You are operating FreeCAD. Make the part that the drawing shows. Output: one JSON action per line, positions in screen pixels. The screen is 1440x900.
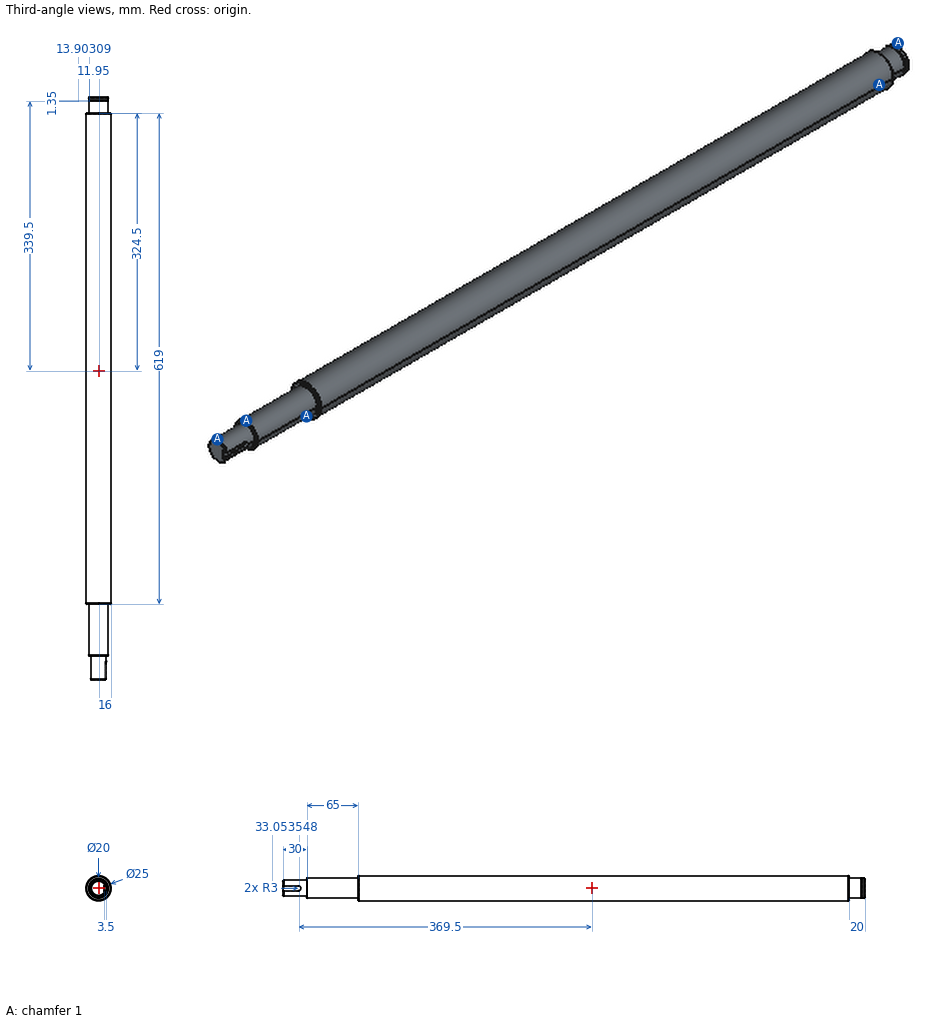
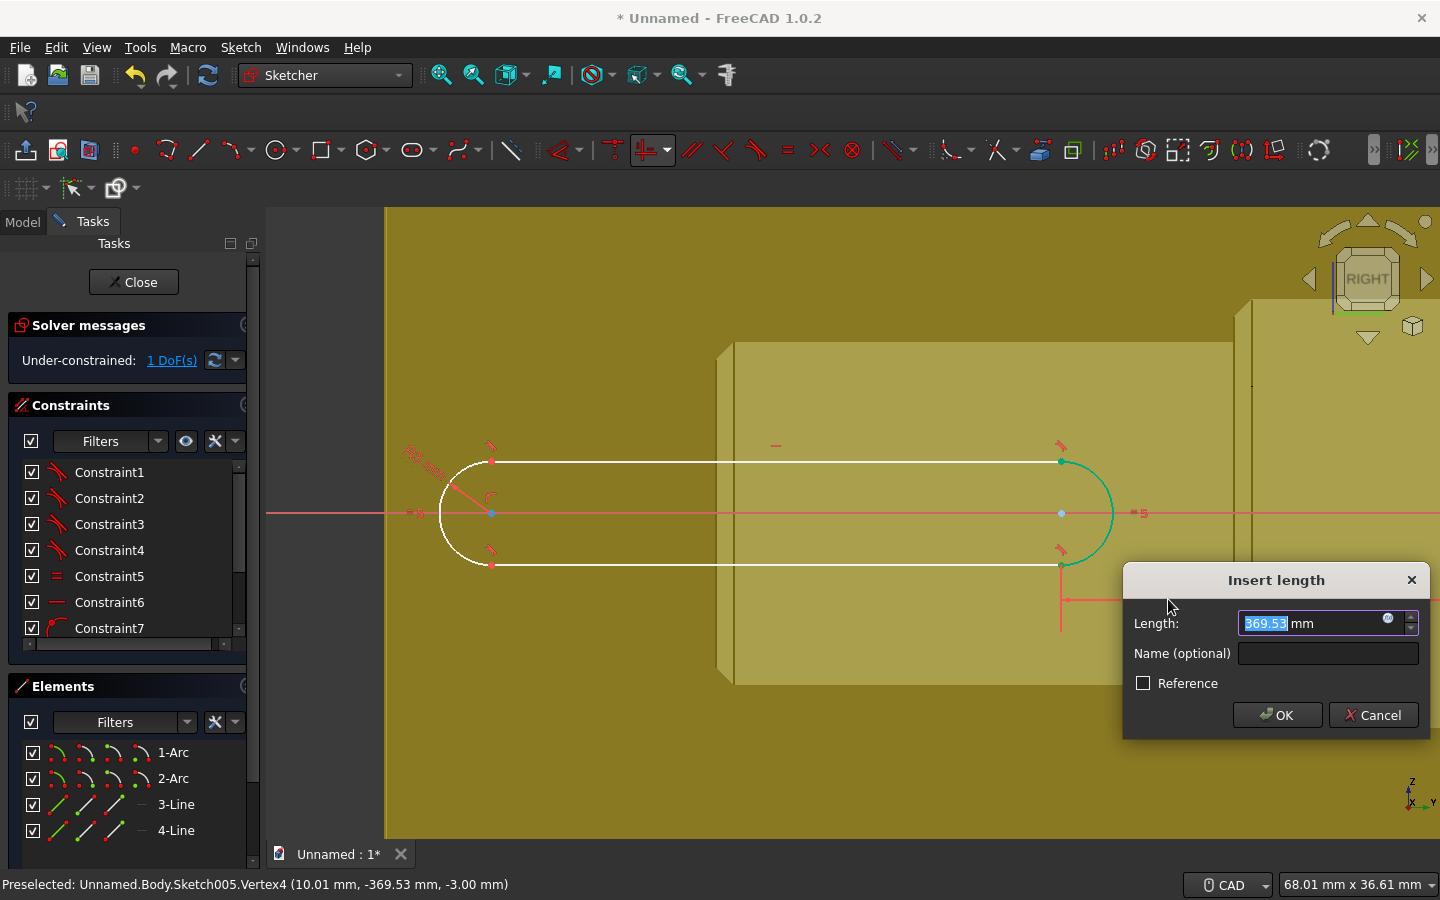
{"action": "type", "text": "369.5"}
{"action": "key", "text": "Return"}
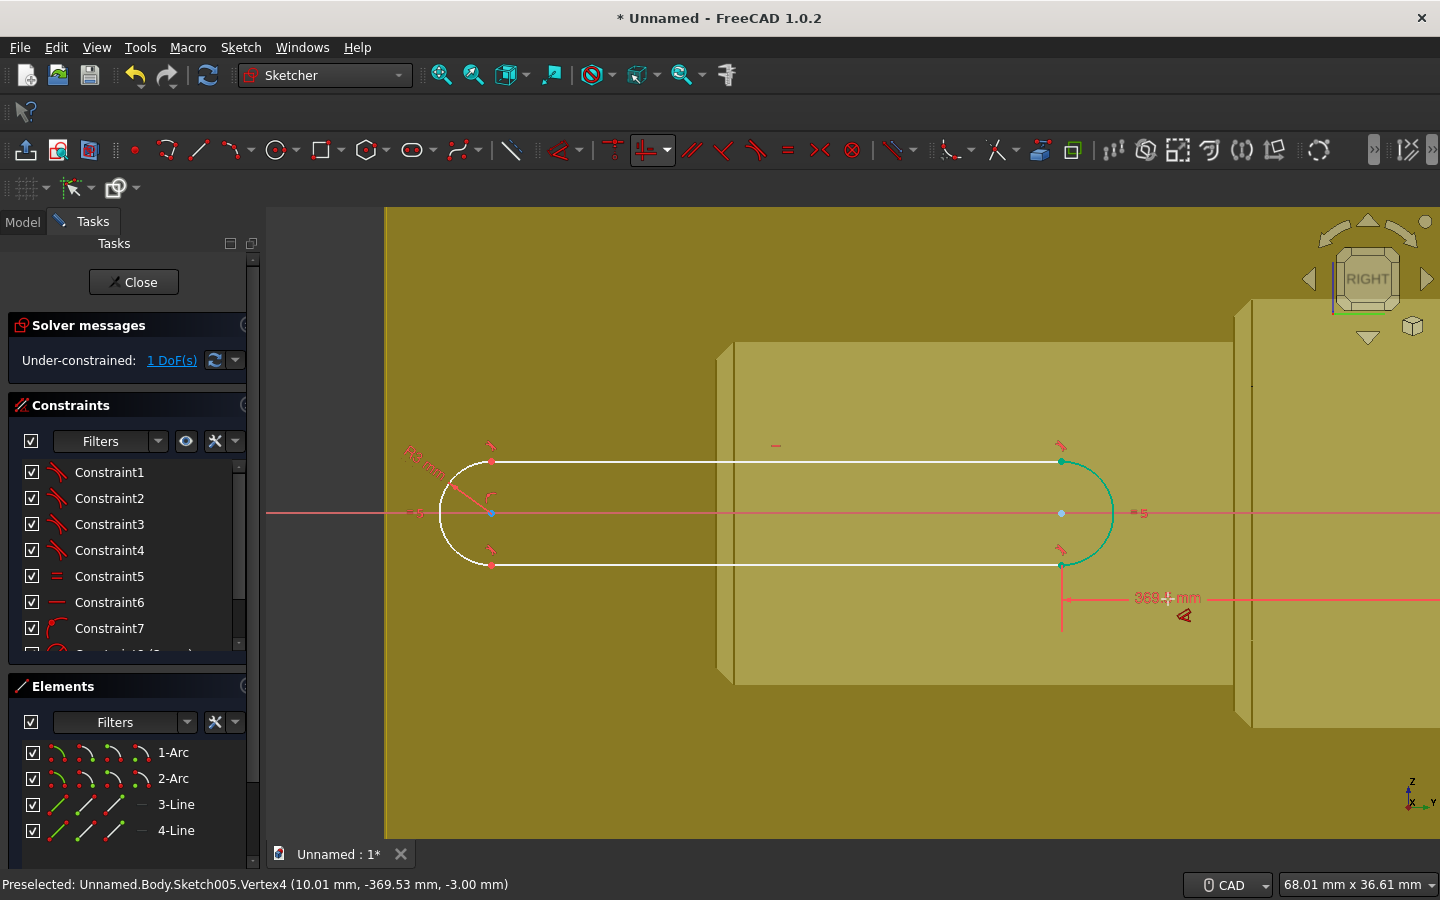
{"action": "left_click", "coordinate": [662, 462]}
{"action": "left_click", "coordinate": [776, 428]}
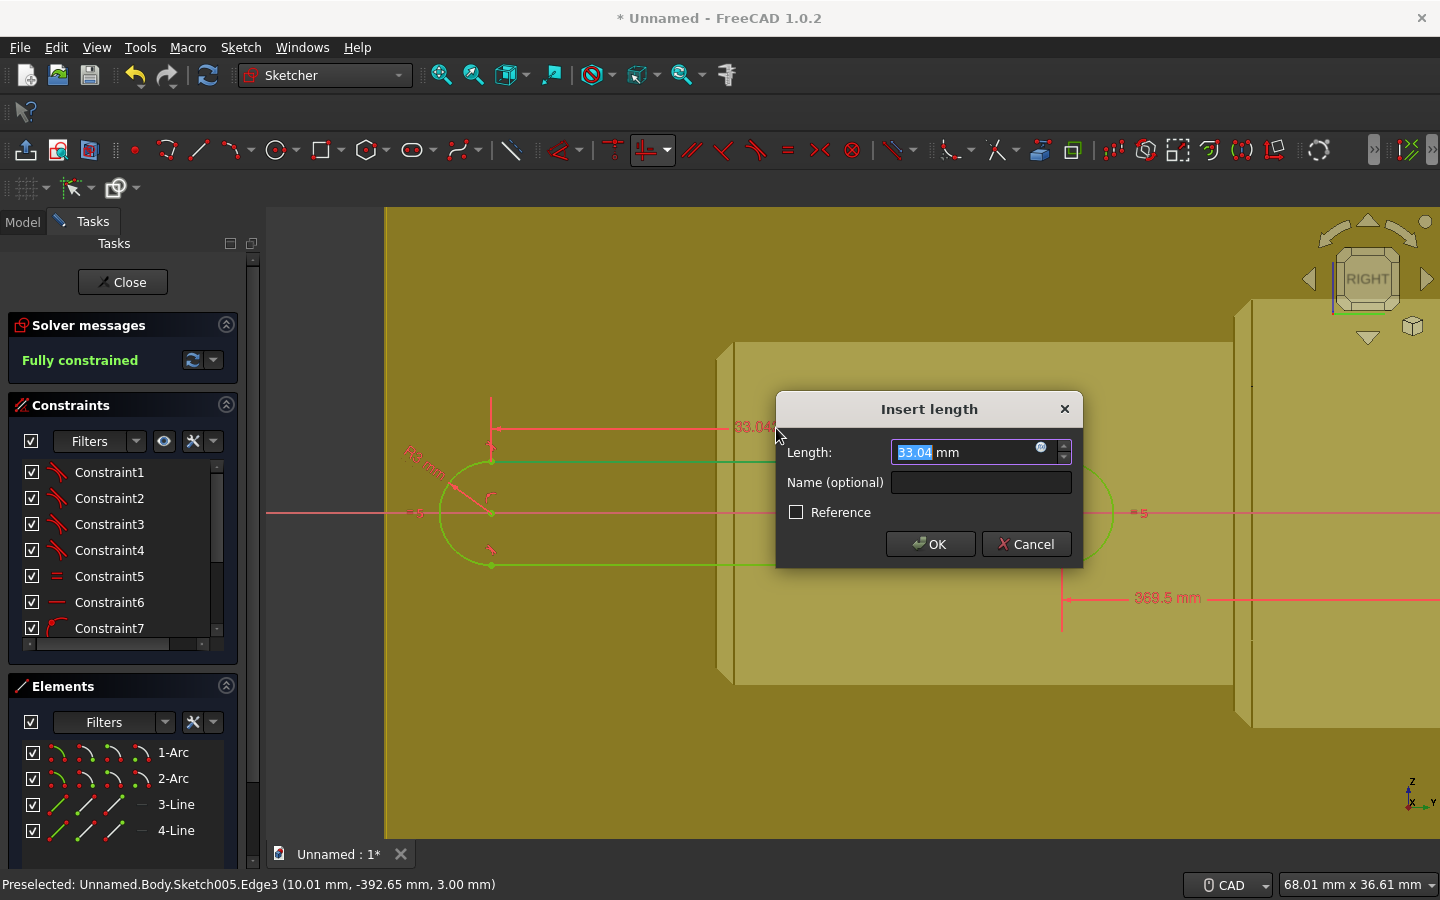
{"action": "type", "text": "33.053548"}
{"action": "key", "text": "Return"}
{"action": "key", "text": "Escape"}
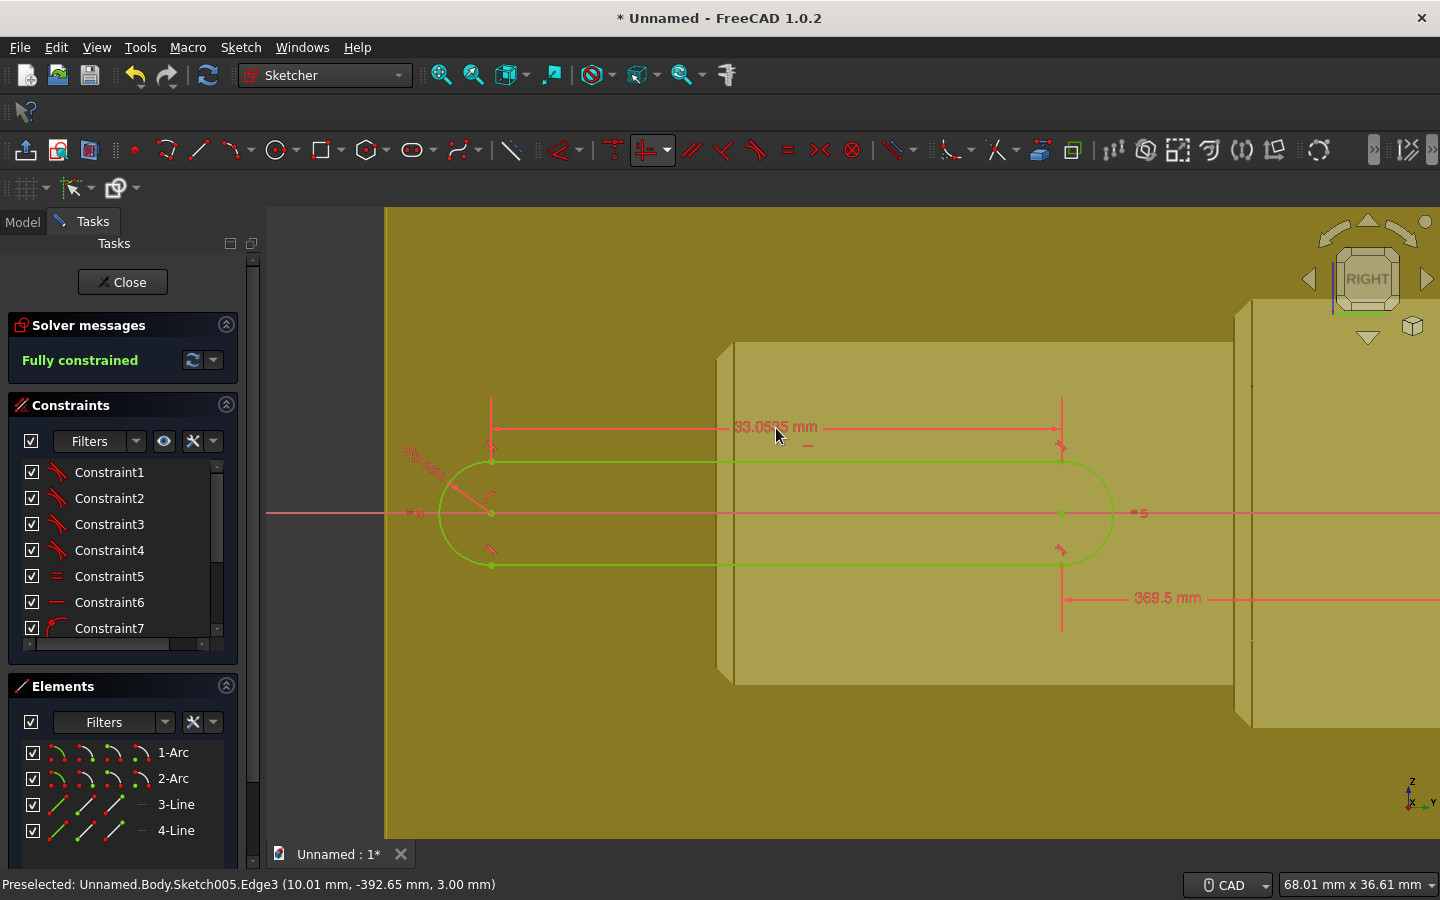
{"action": "left_click", "coordinate": [123, 282]}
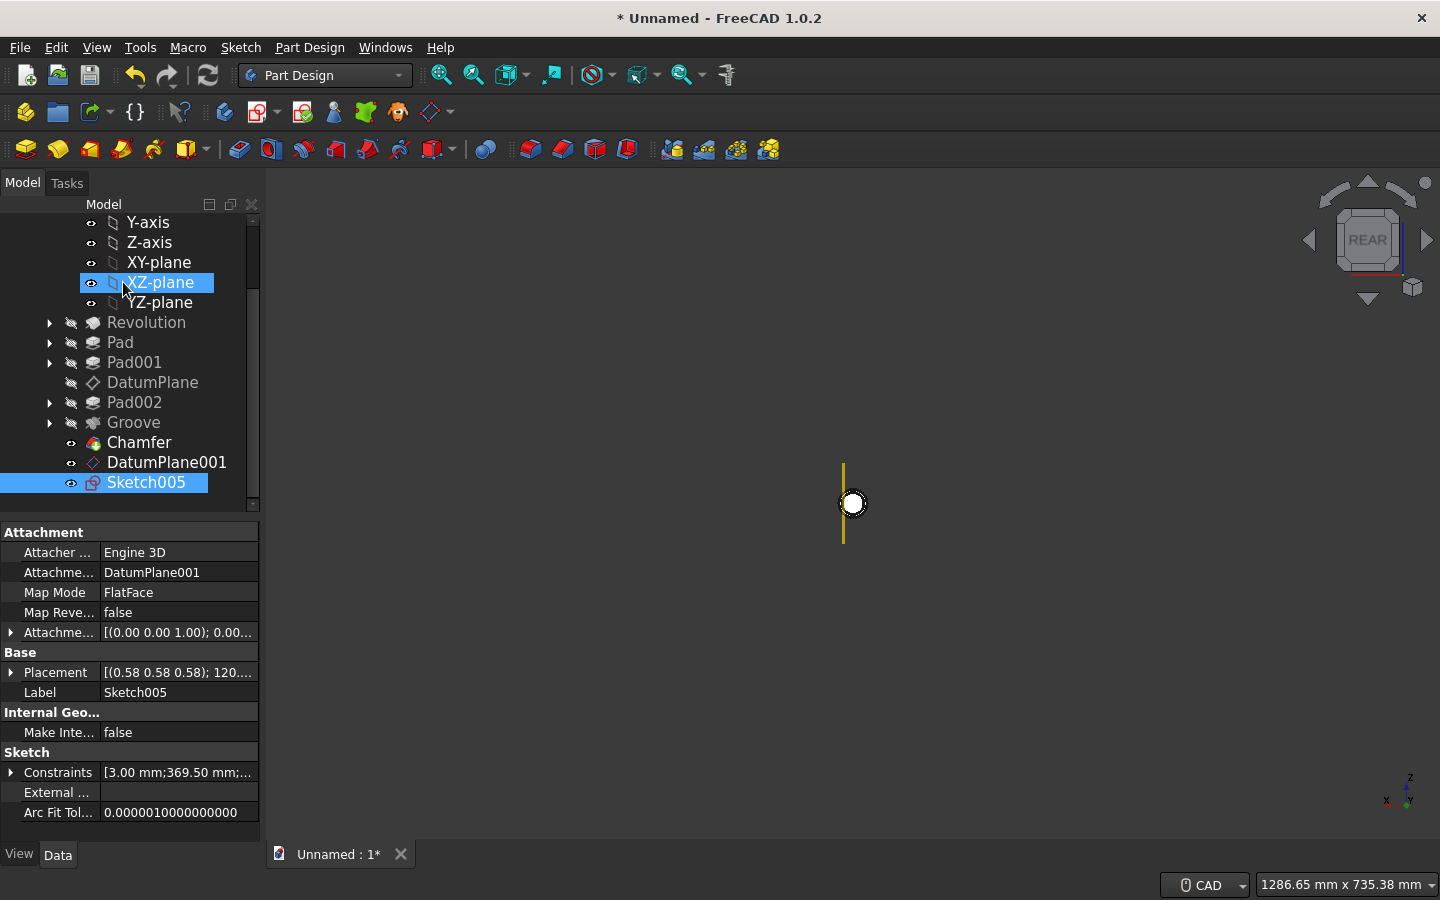
{"action": "left_click", "coordinate": [240, 150]}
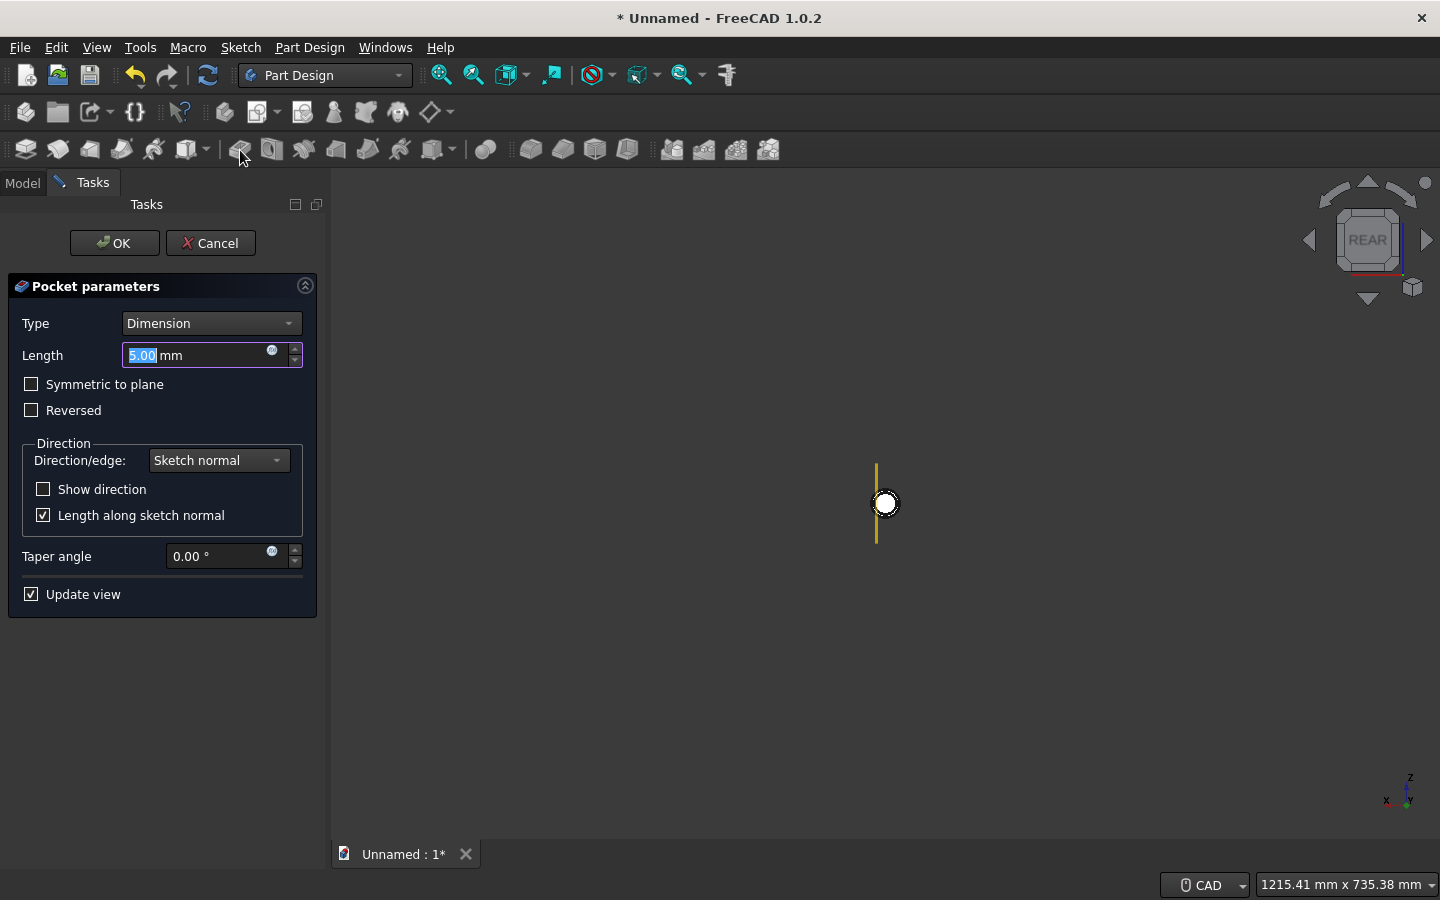
{"action": "type", "text": "3.5"}
{"action": "key", "text": "Tab"}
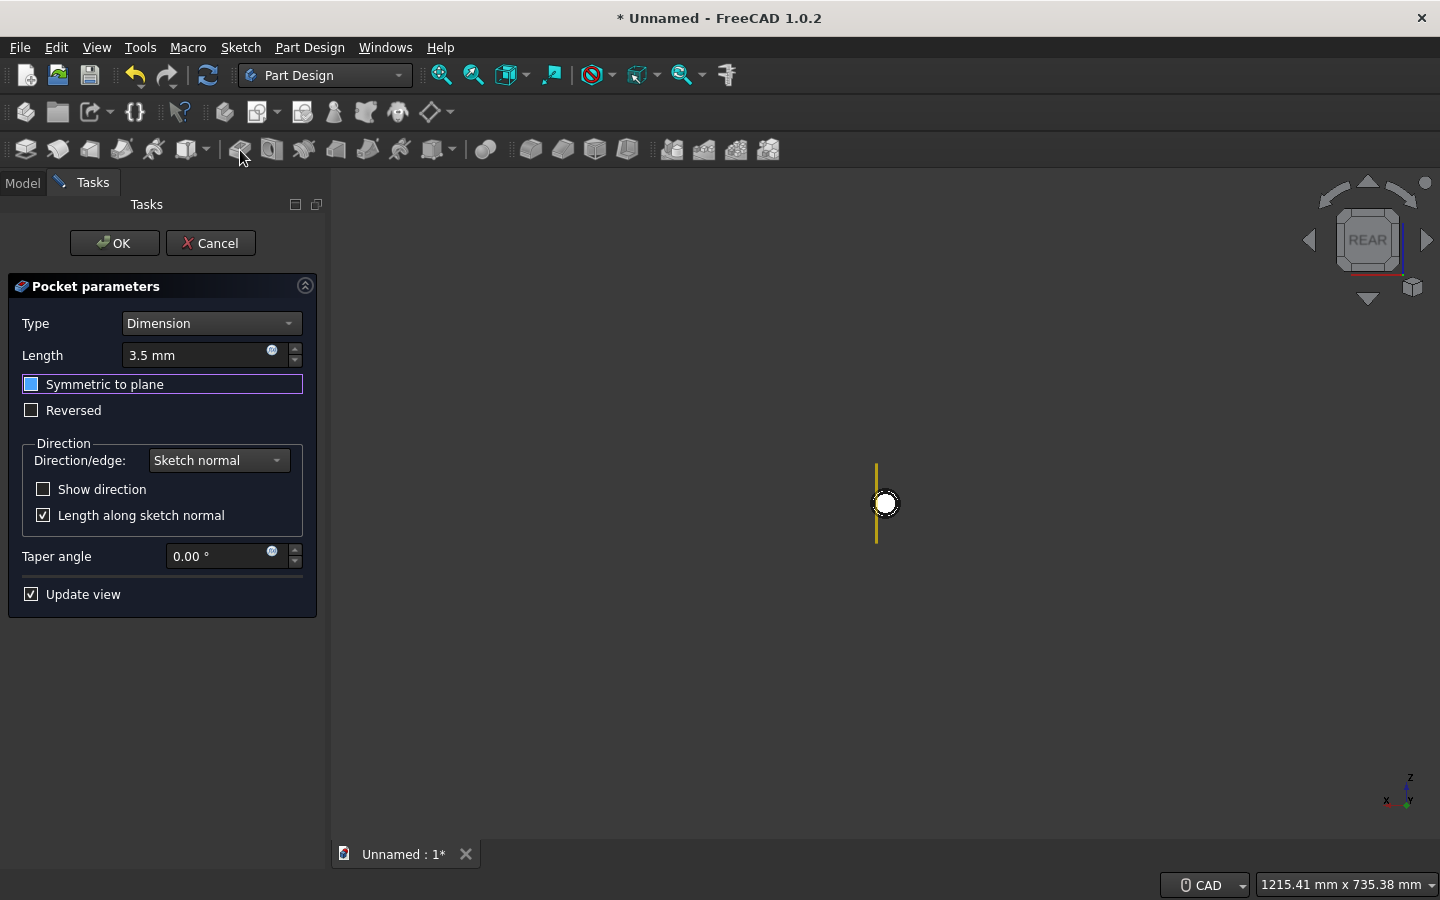
{"action": "left_click", "coordinate": [115, 243]}